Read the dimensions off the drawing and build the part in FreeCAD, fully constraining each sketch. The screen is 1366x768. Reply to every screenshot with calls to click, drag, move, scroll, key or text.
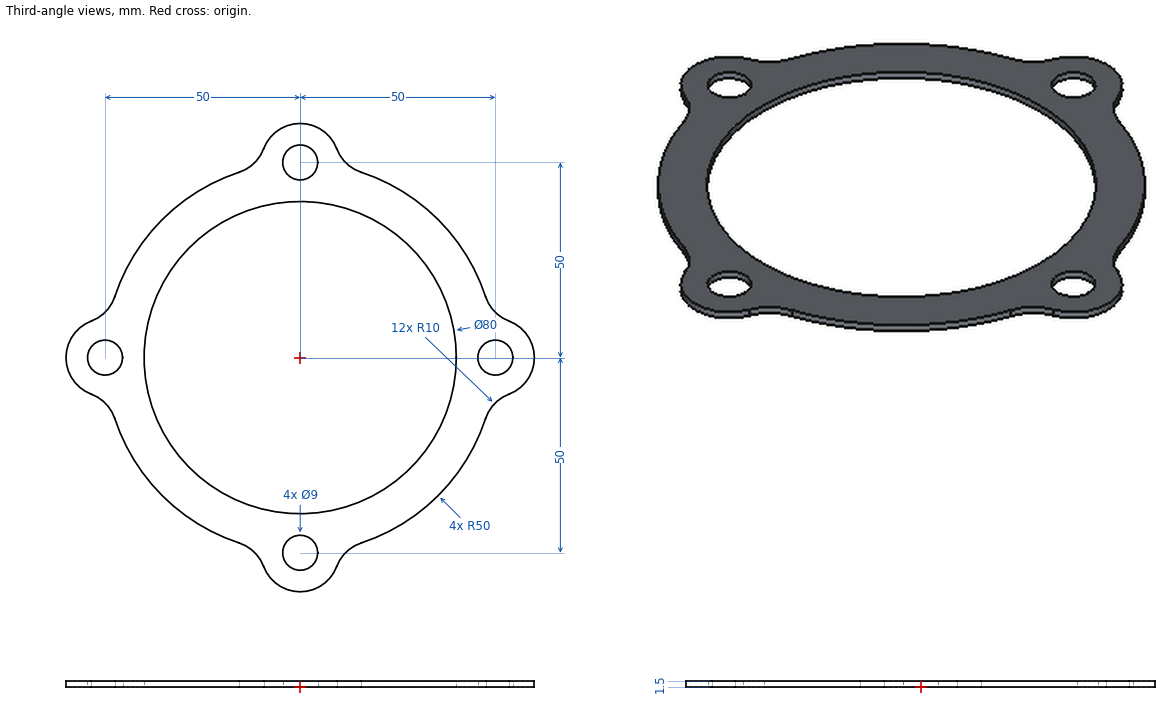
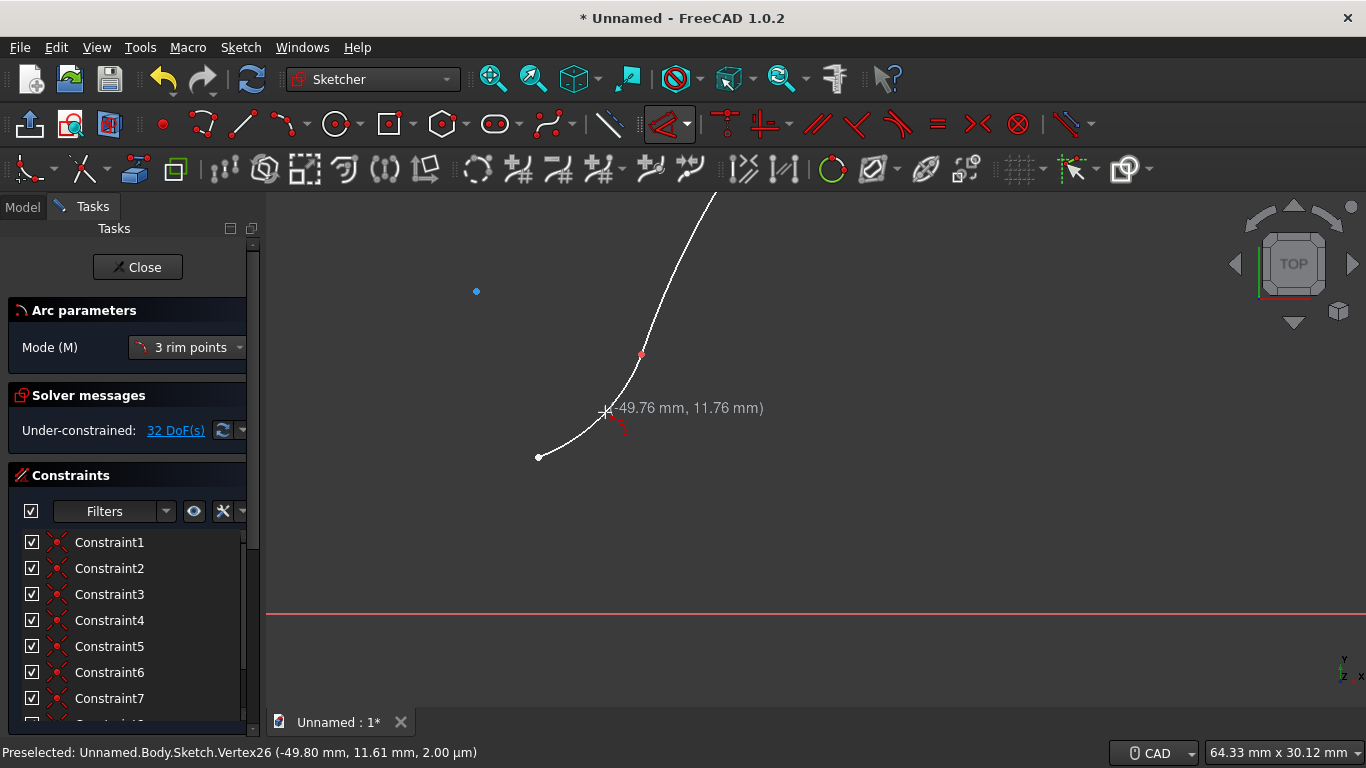
scroll(607, 417, down, 9)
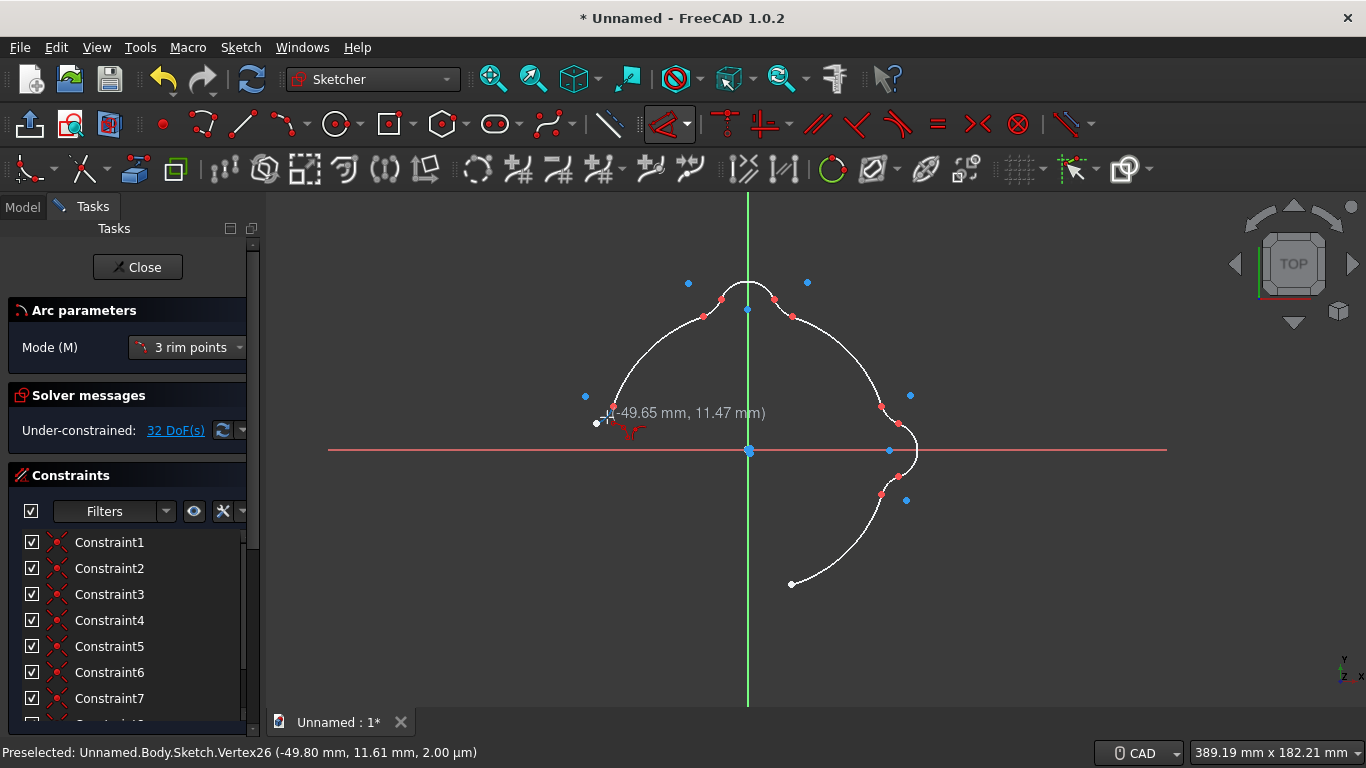
click(596, 424)
click(596, 476)
click(581, 437)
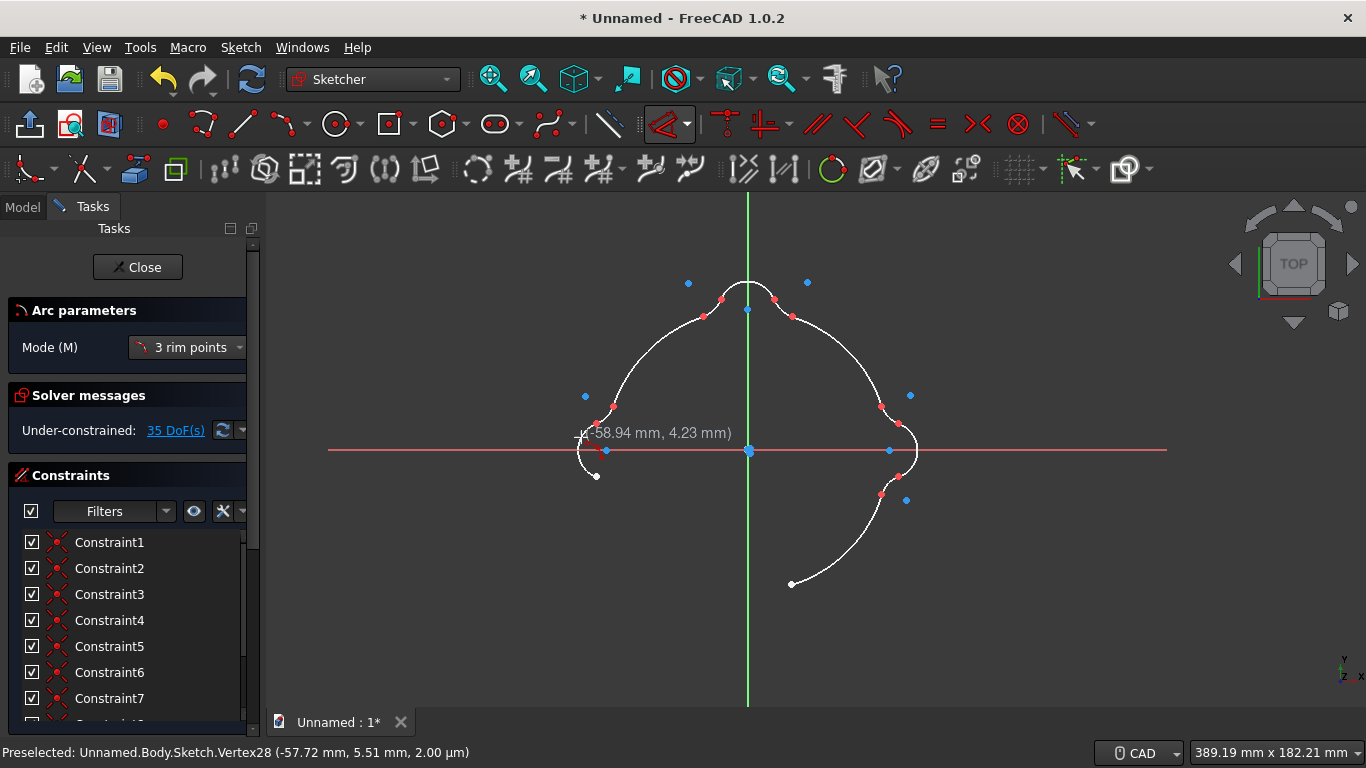
click(596, 477)
click(613, 494)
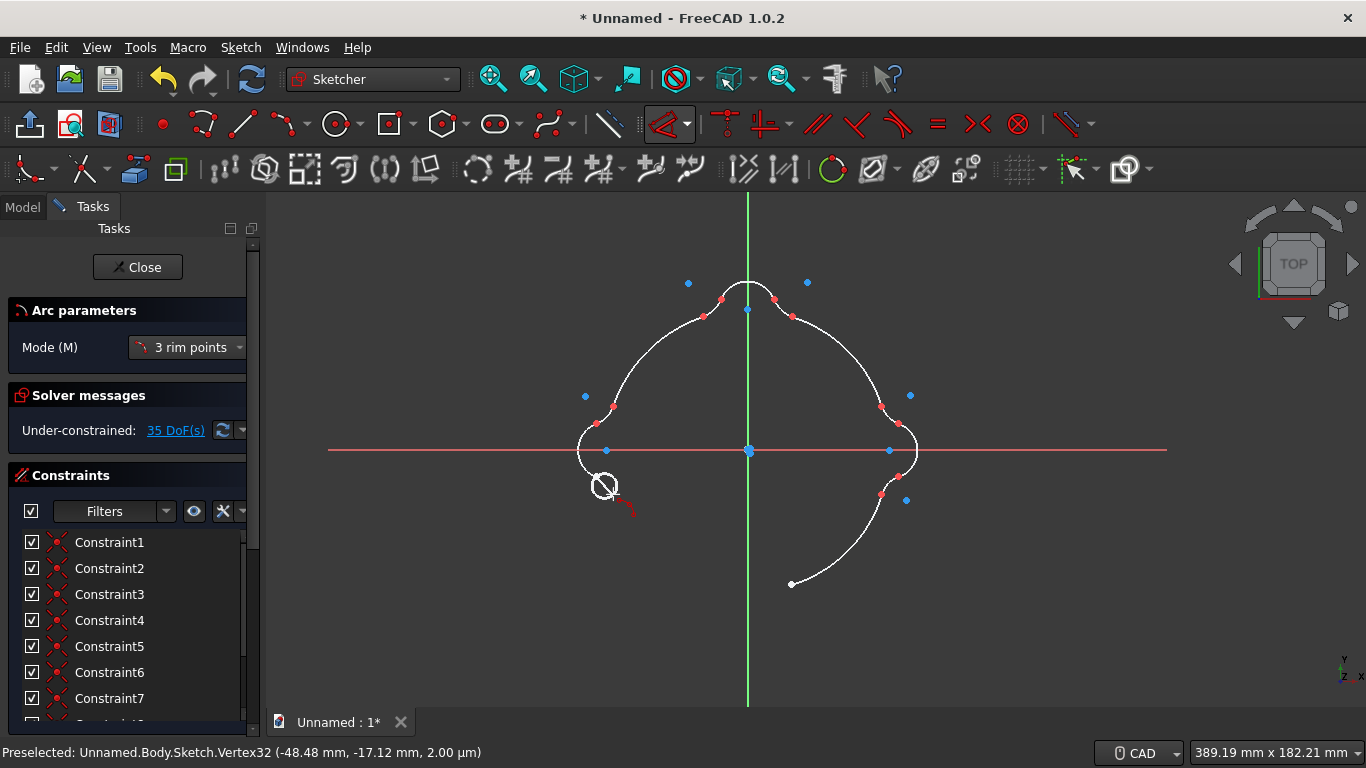
scroll(607, 483, up, 9)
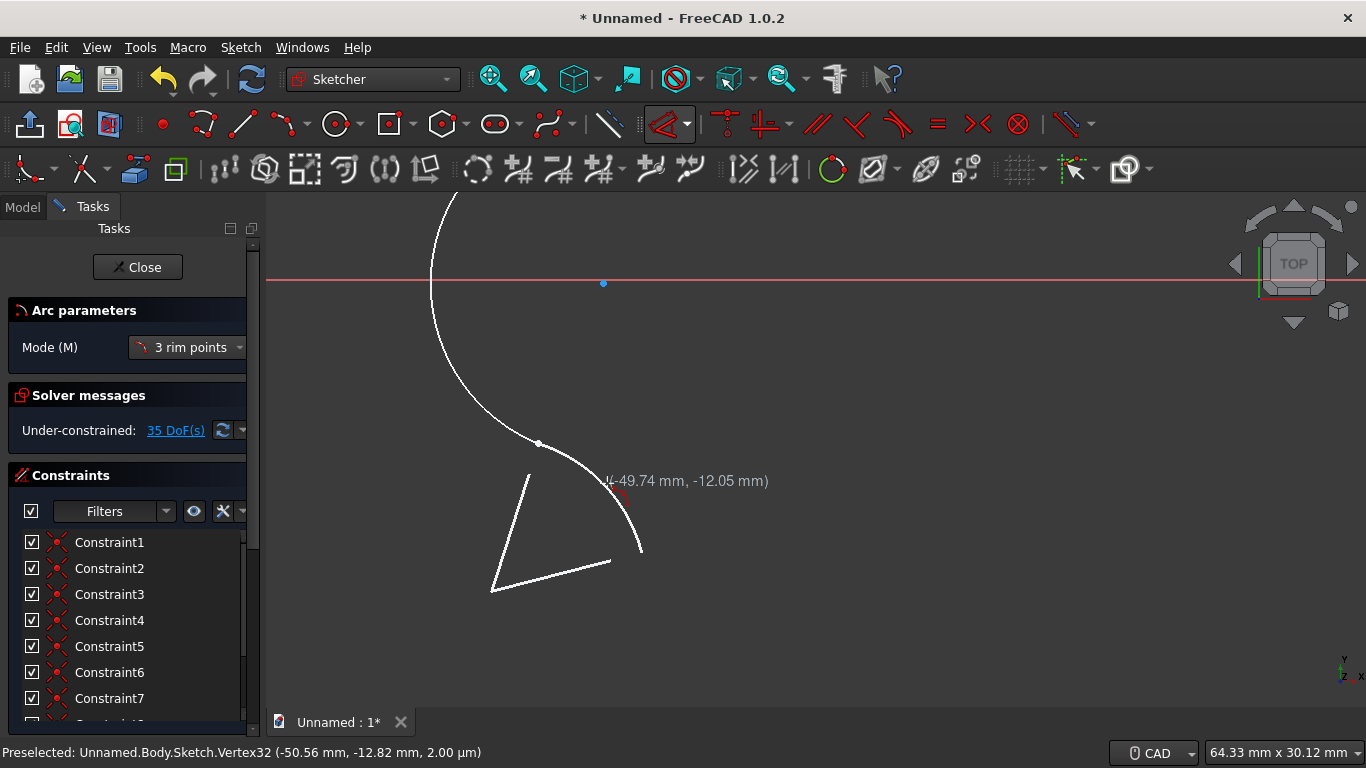
click(605, 482)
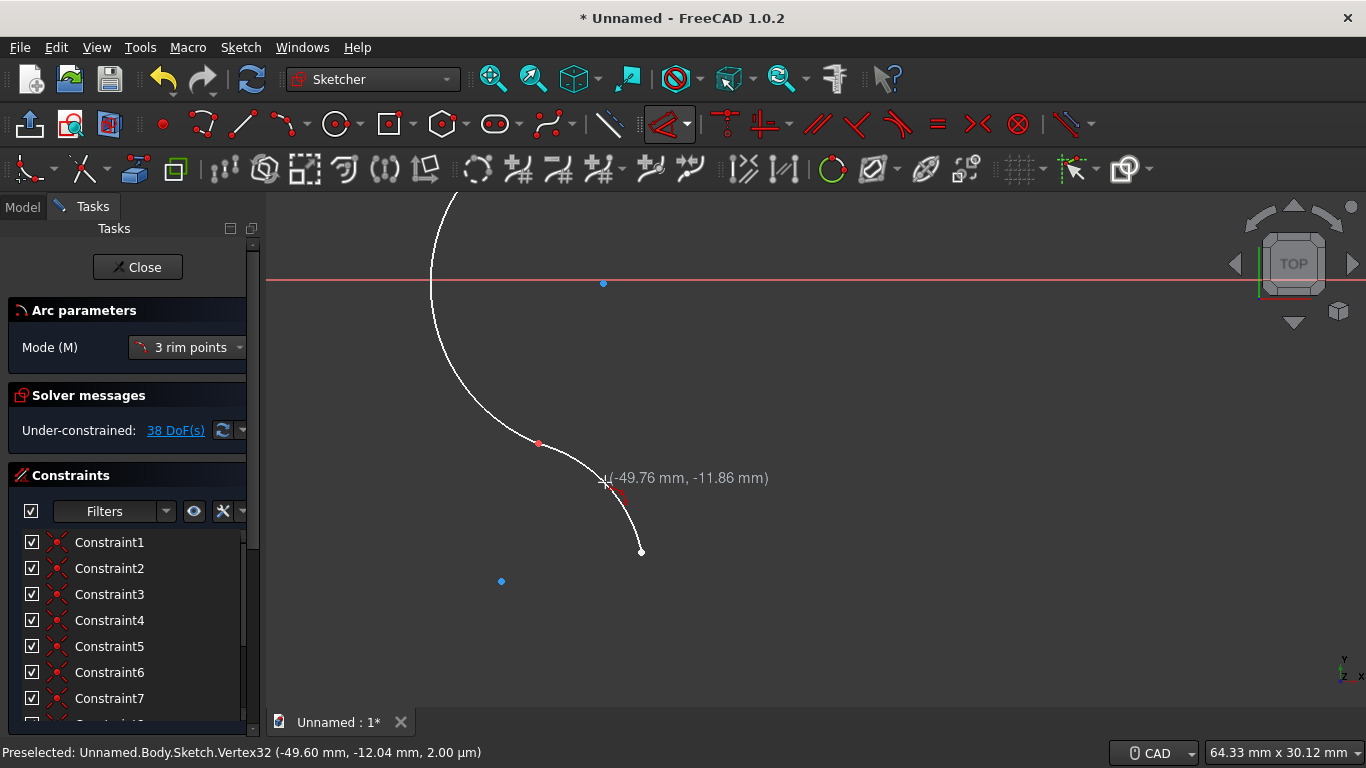
scroll(607, 483, down, 9)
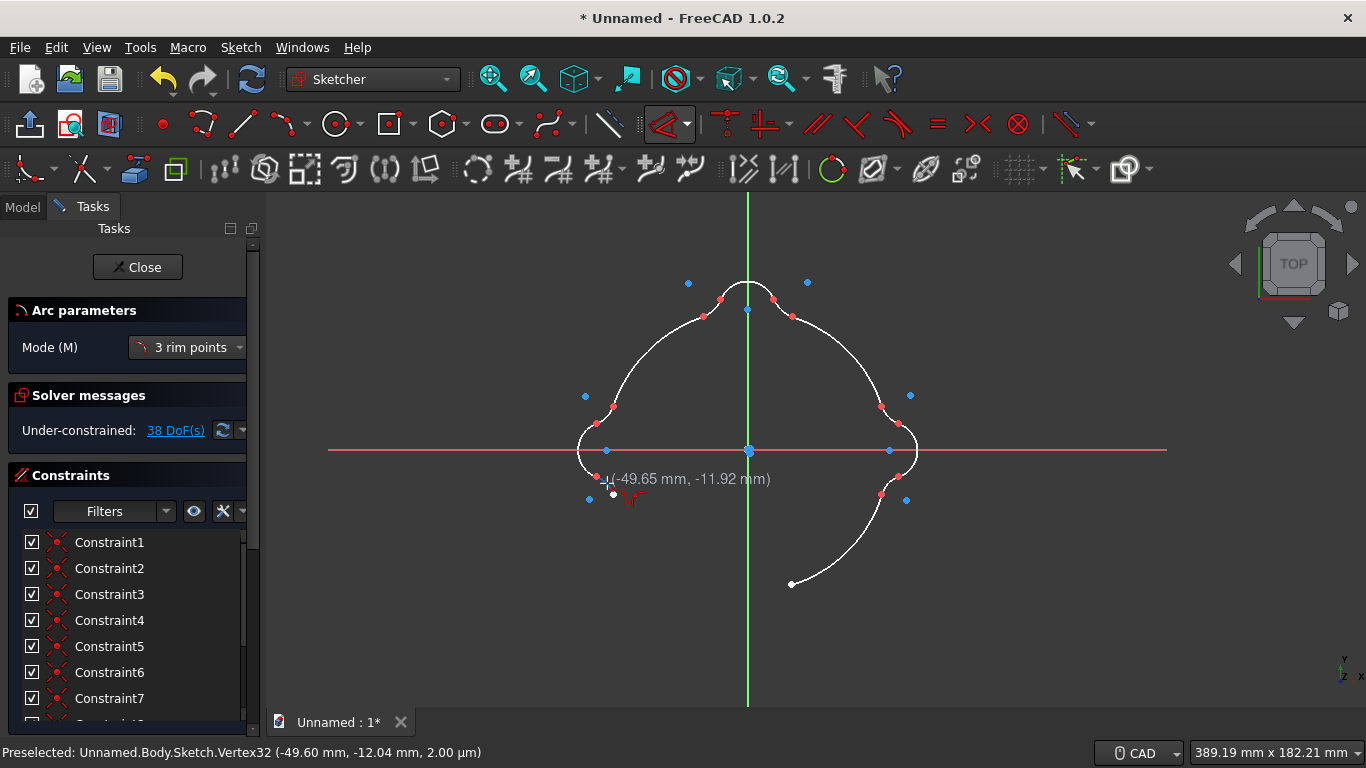
click(613, 495)
click(703, 584)
click(648, 550)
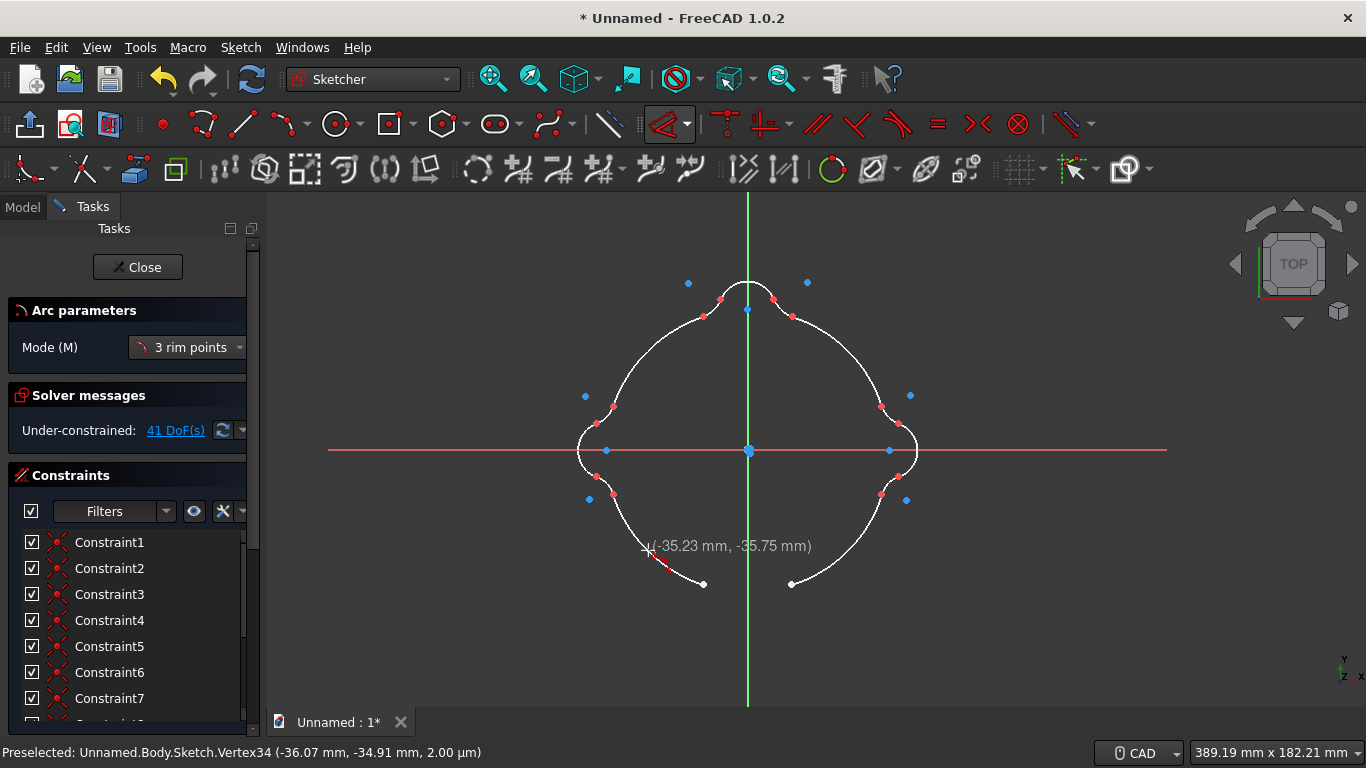
click(703, 585)
click(721, 601)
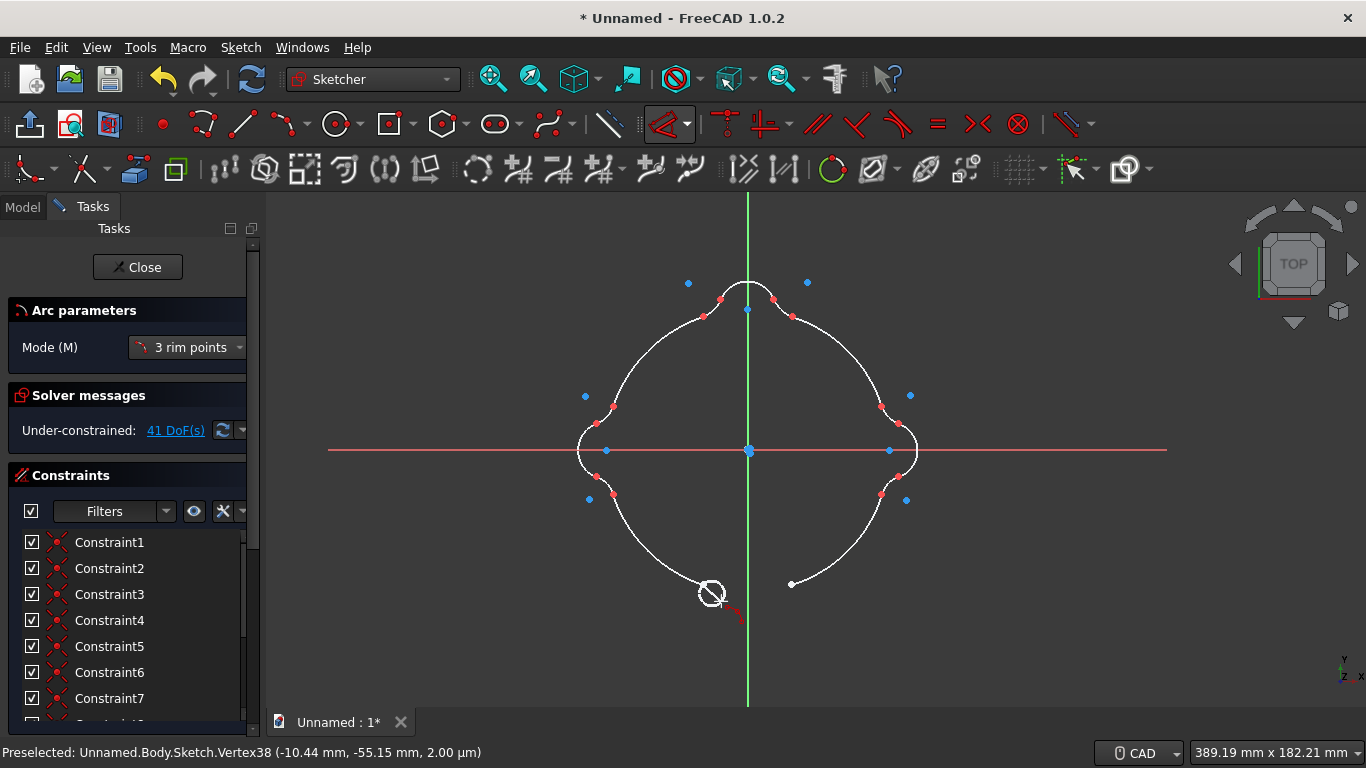
scroll(714, 591, up, 9)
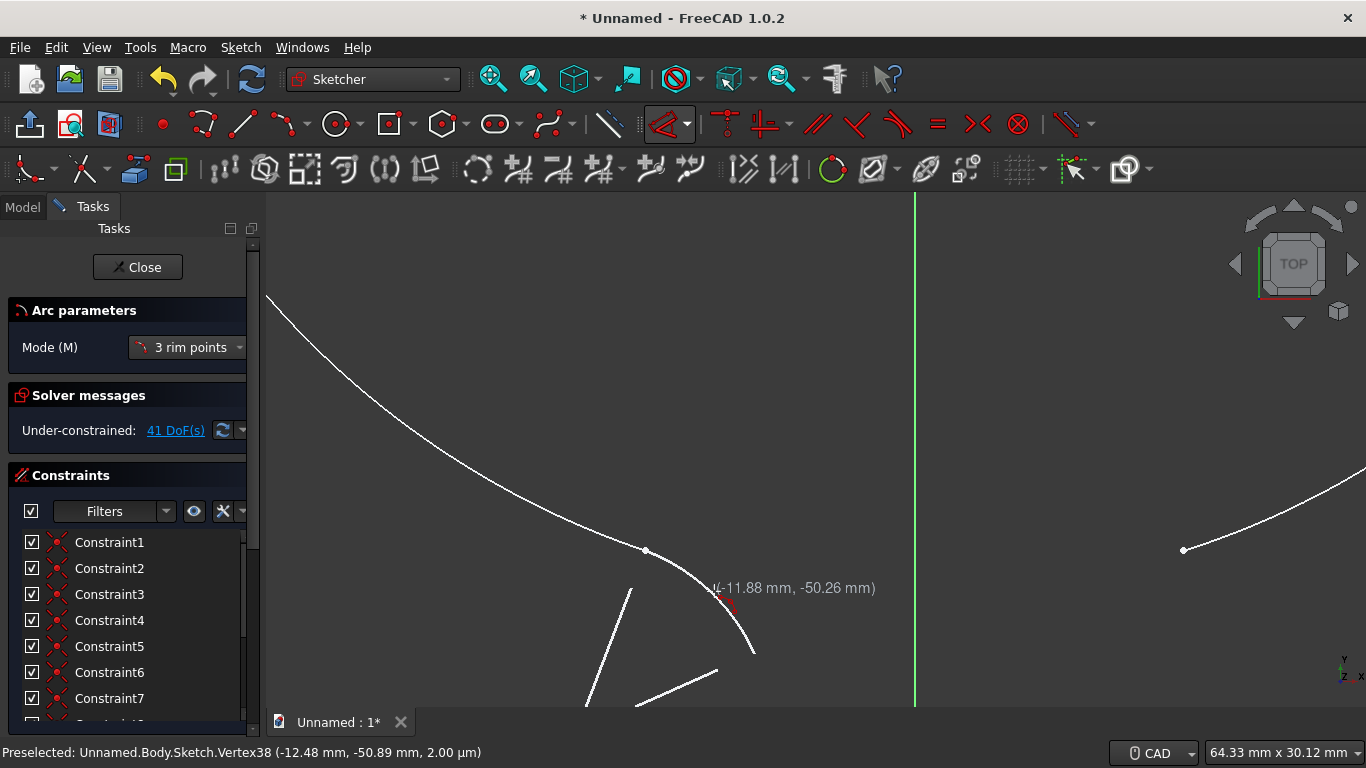
click(713, 585)